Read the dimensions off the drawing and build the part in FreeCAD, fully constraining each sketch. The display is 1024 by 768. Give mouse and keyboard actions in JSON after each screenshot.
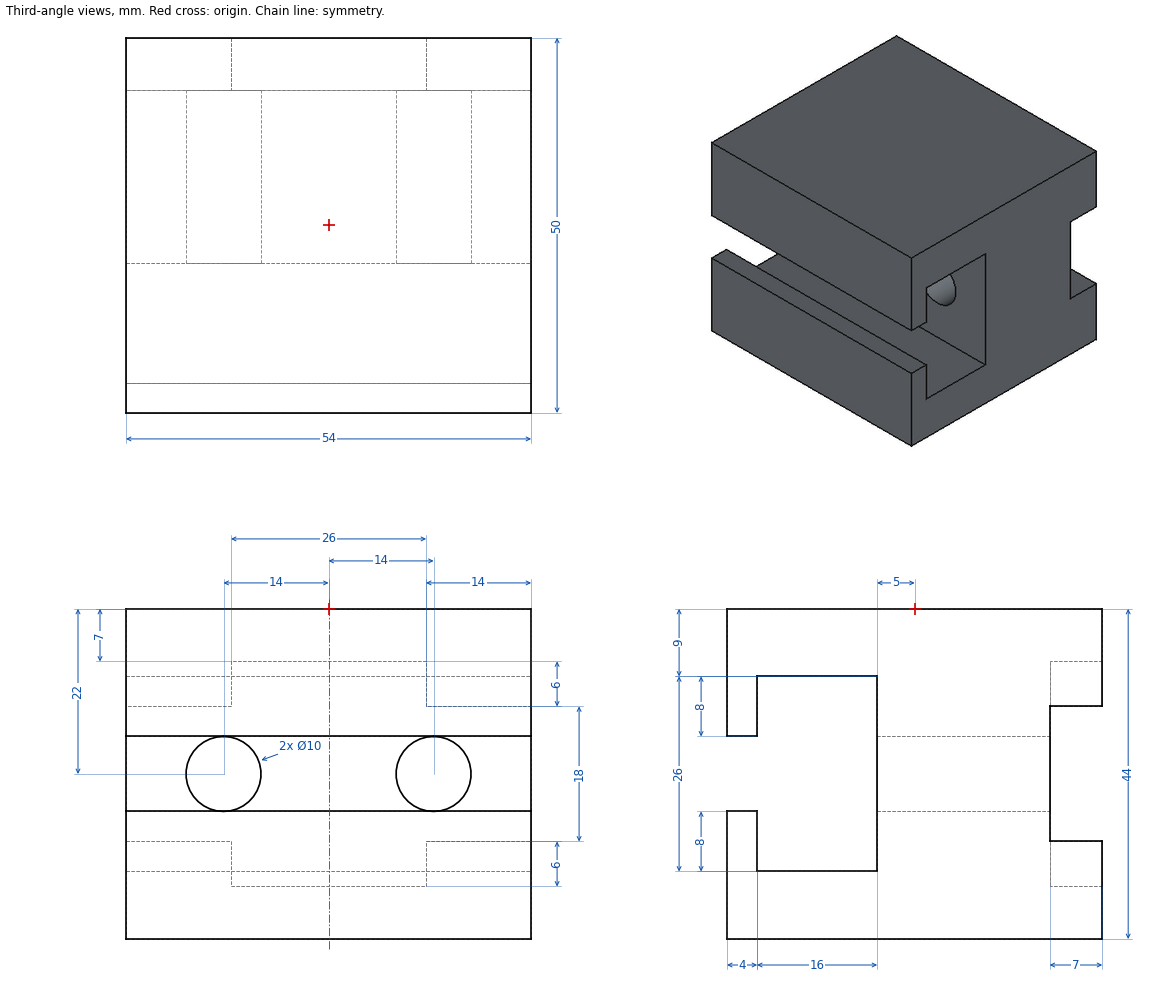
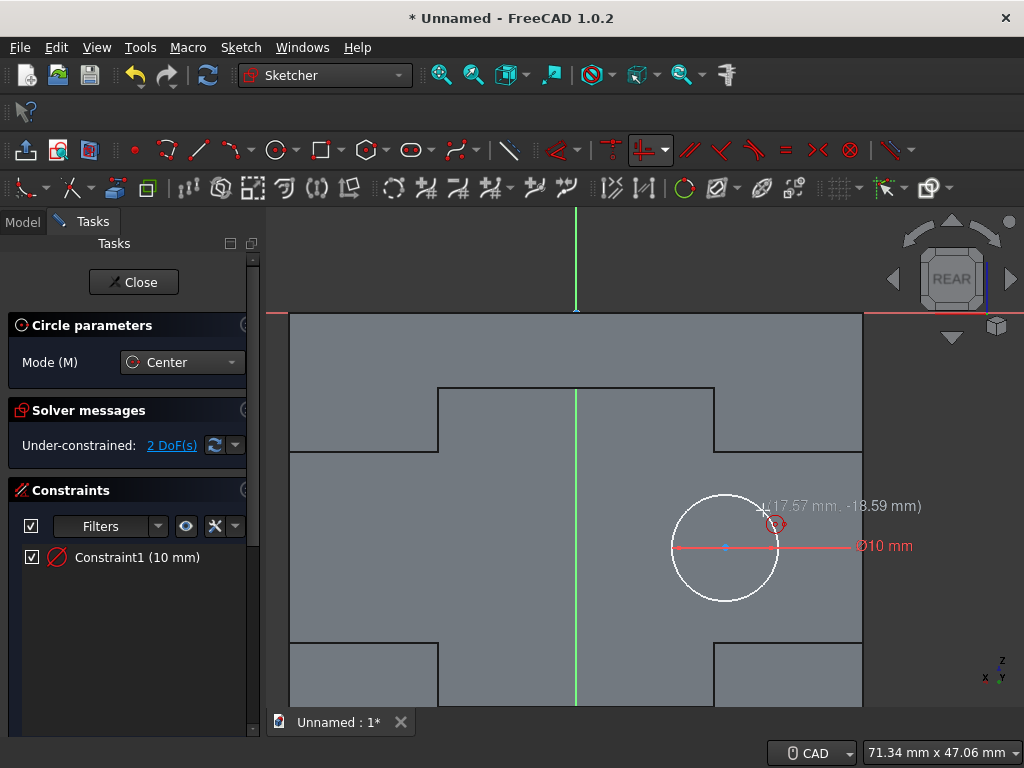
{"action": "left_click", "coordinate": [428, 547]}
{"action": "mouse_move", "coordinate": [465, 510]}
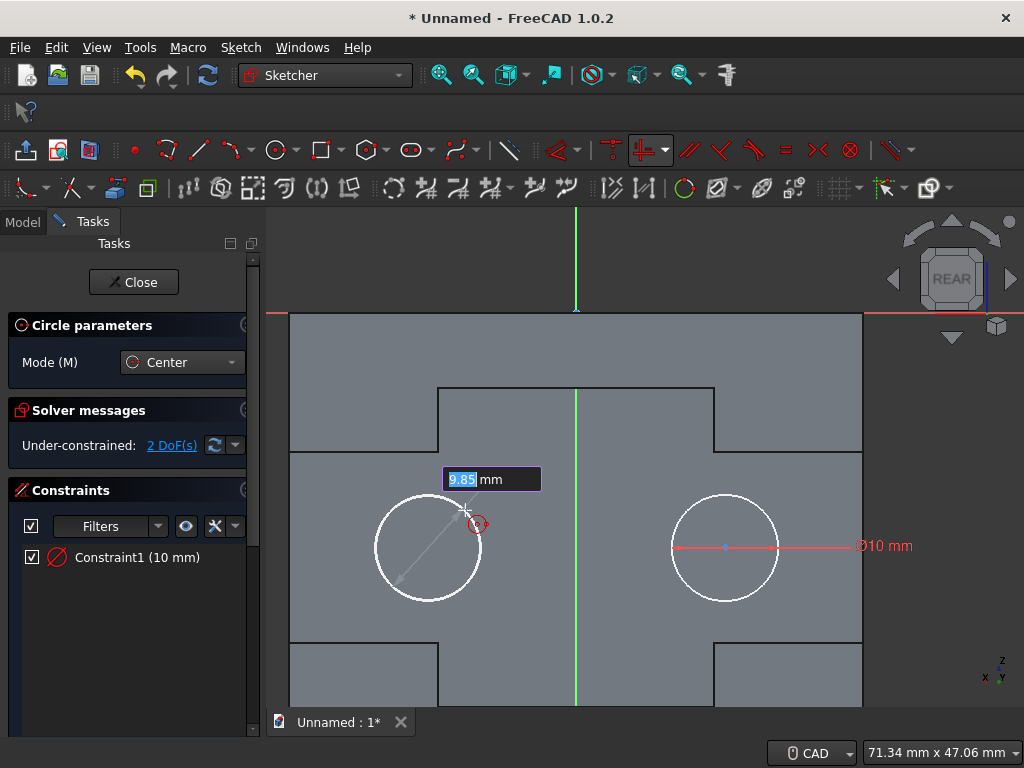
{"action": "type", "text": "10"}
{"action": "key", "text": "Return"}
{"action": "key", "text": "Escape"}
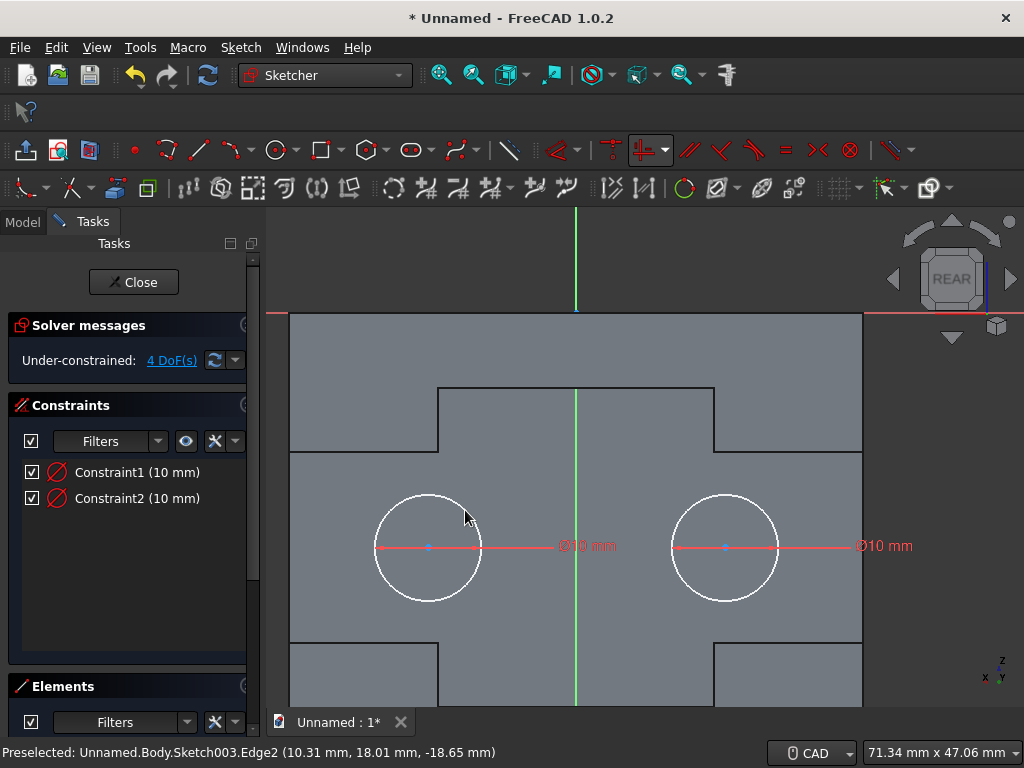
{"action": "left_click", "coordinate": [725, 548]}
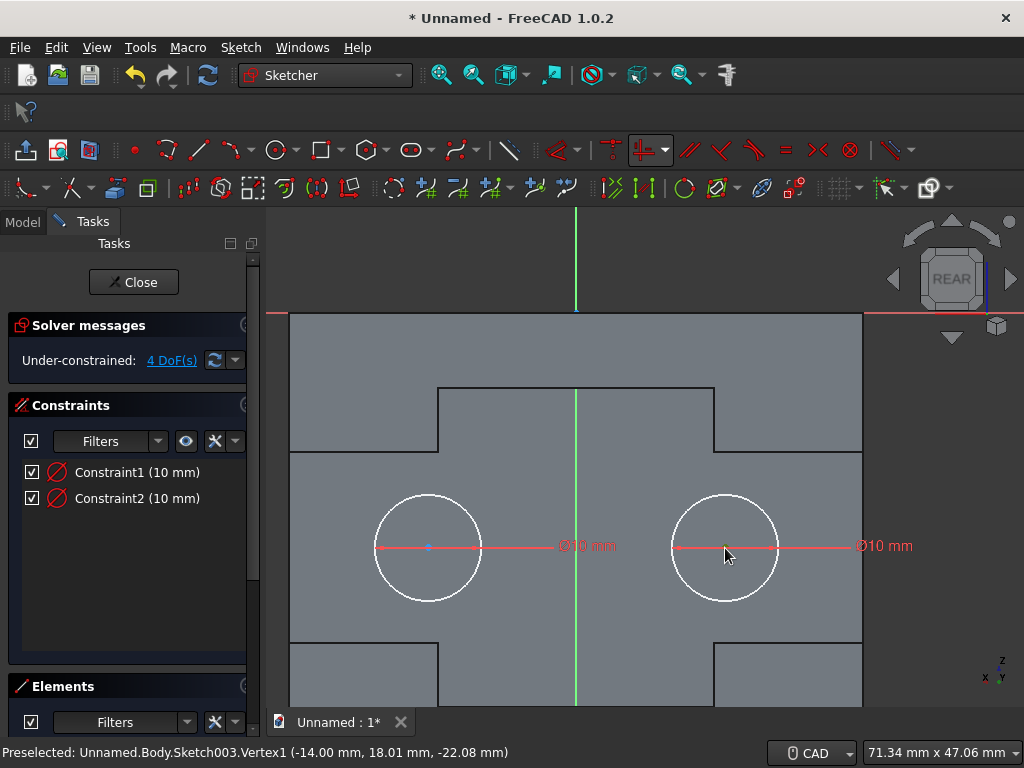
{"action": "left_click", "coordinate": [428, 548]}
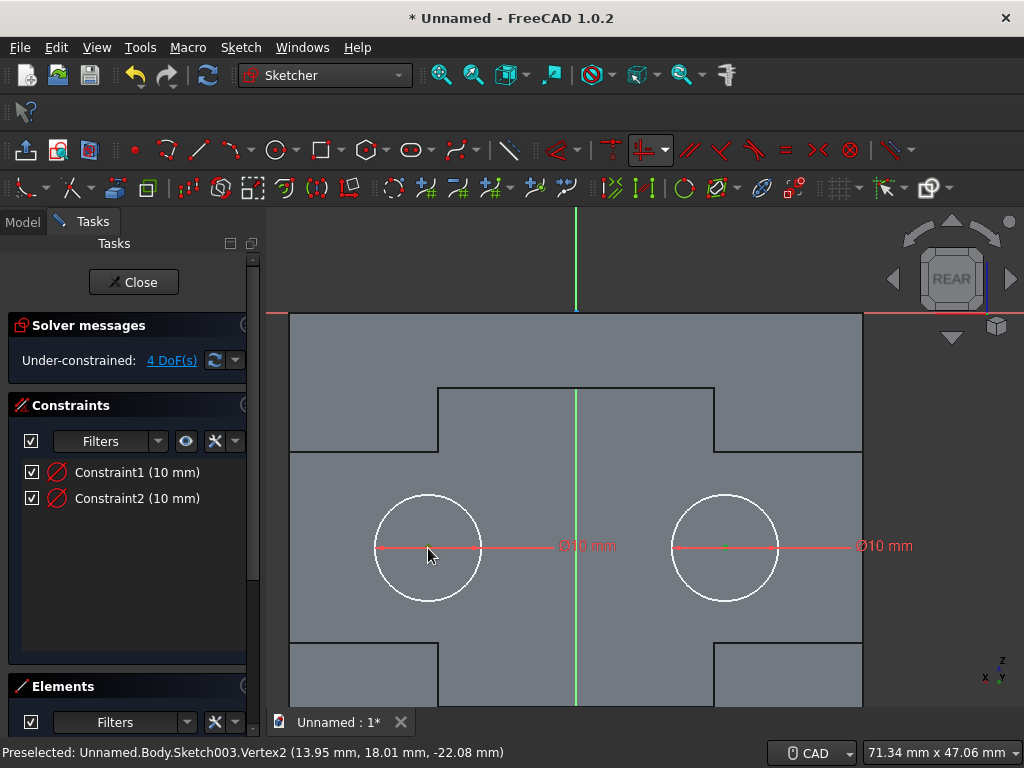
{"action": "key", "text": "h"}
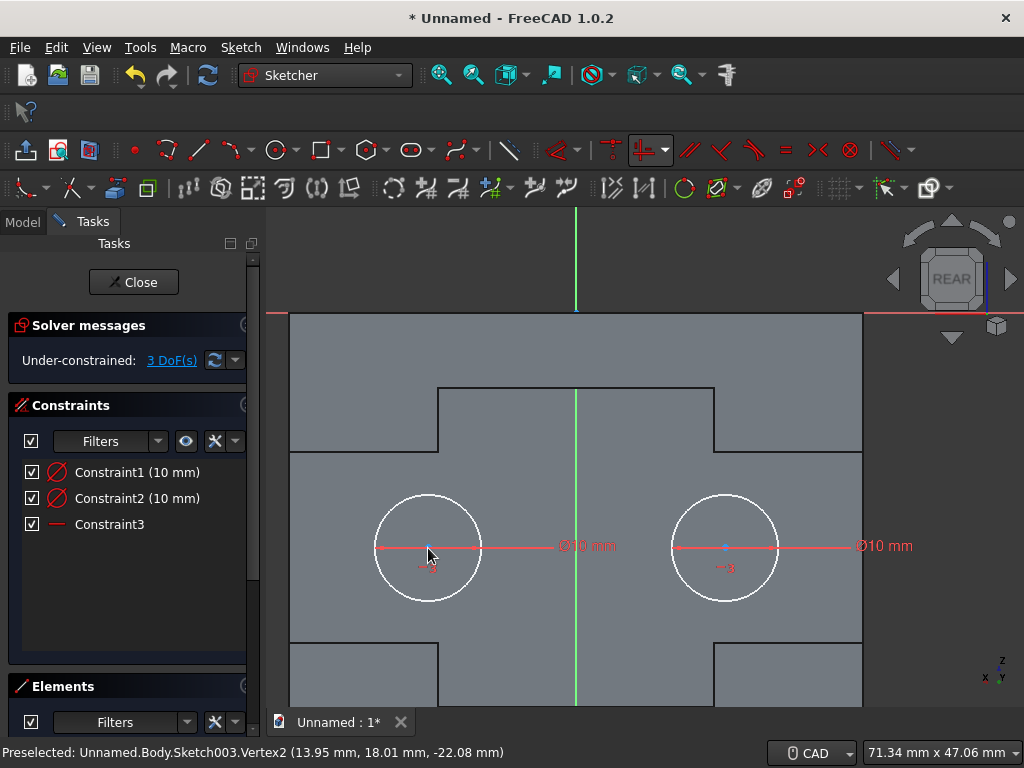
{"action": "left_click", "coordinate": [556, 150]}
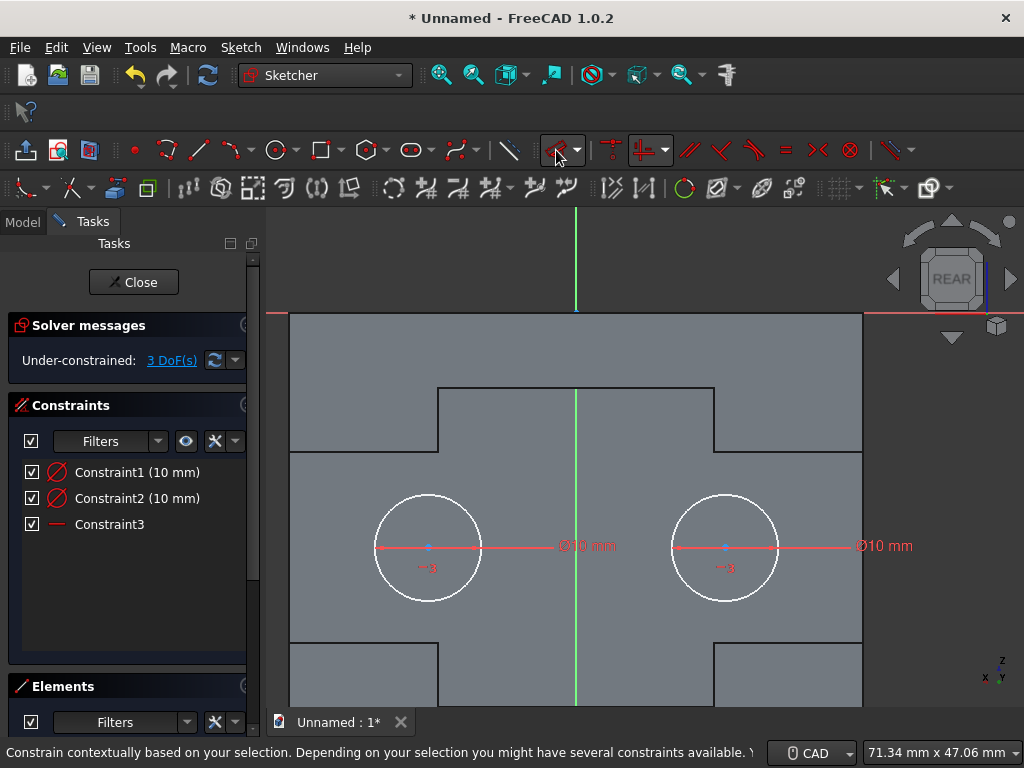
{"action": "left_click", "coordinate": [725, 548]}
{"action": "left_click", "coordinate": [651, 279]}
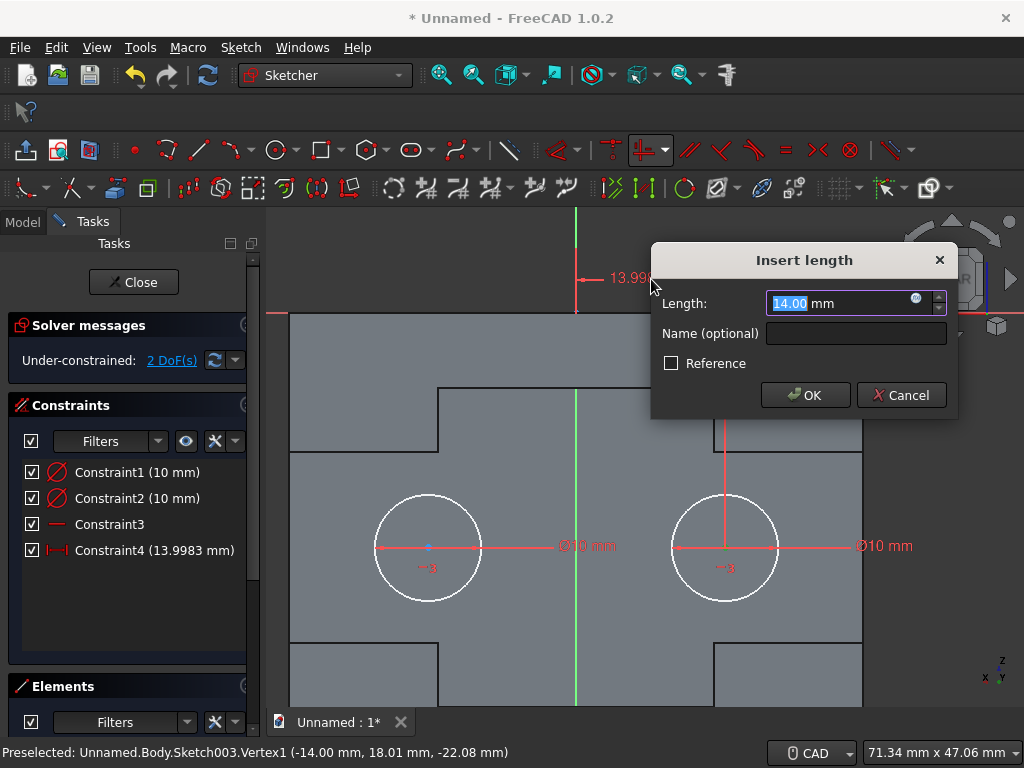
{"action": "type", "text": "14"}
{"action": "key", "text": "Return"}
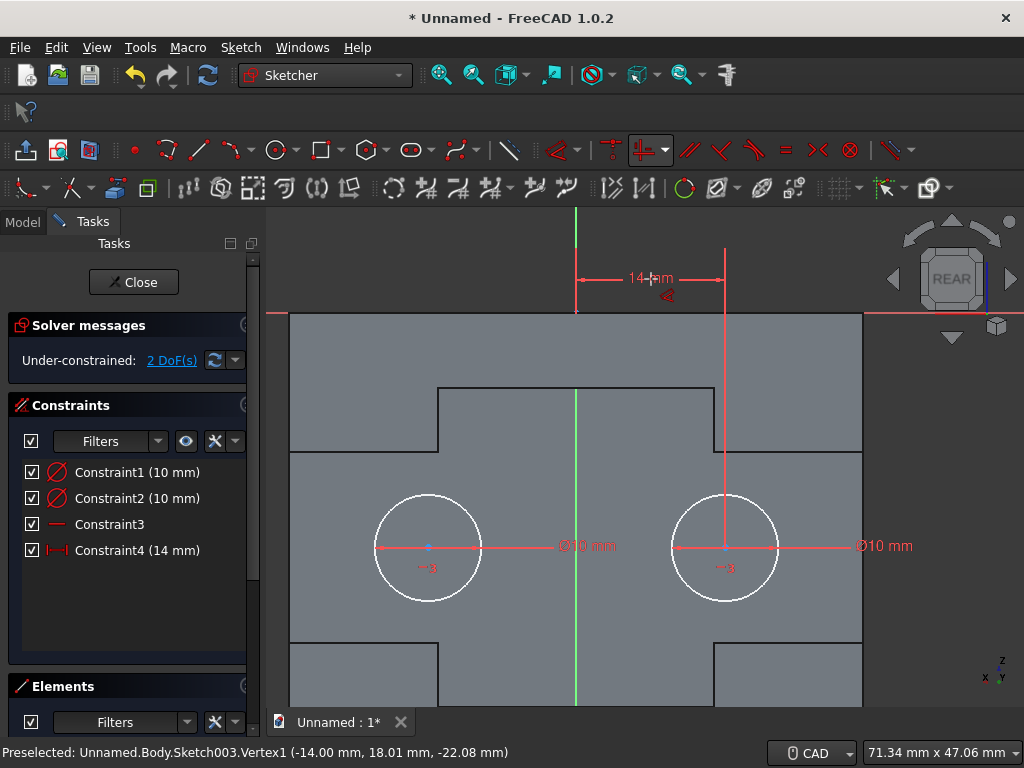
{"action": "left_click", "coordinate": [725, 548]}
{"action": "left_click", "coordinate": [759, 431]}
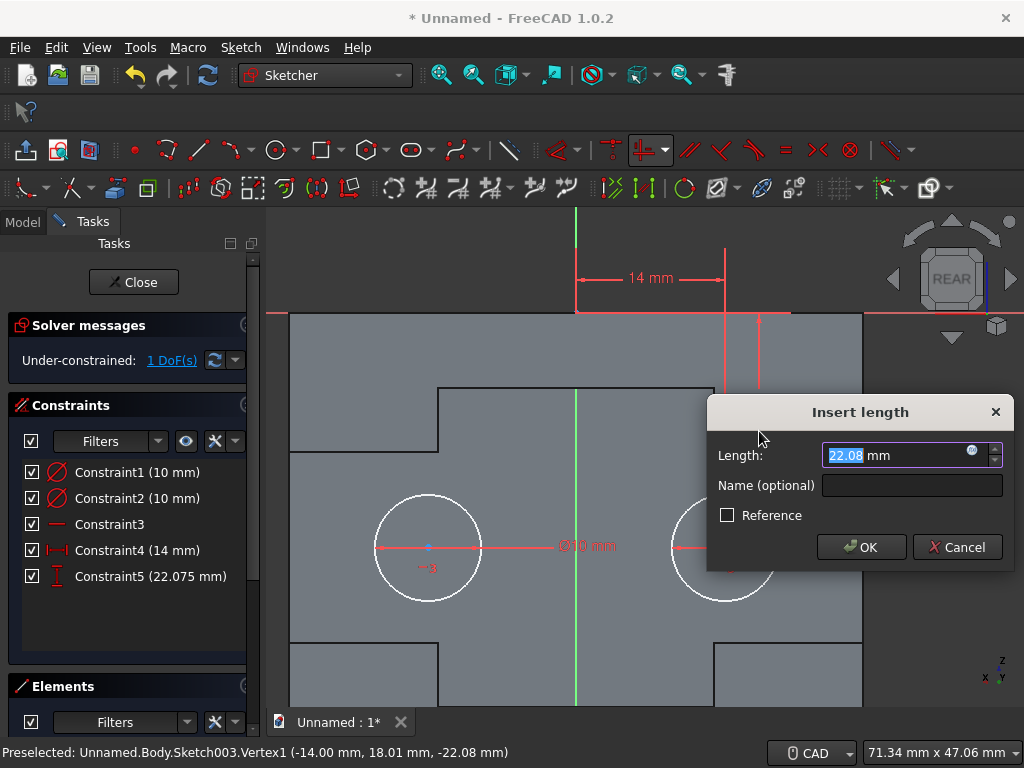
{"action": "type", "text": "22"}
{"action": "key", "text": "Return"}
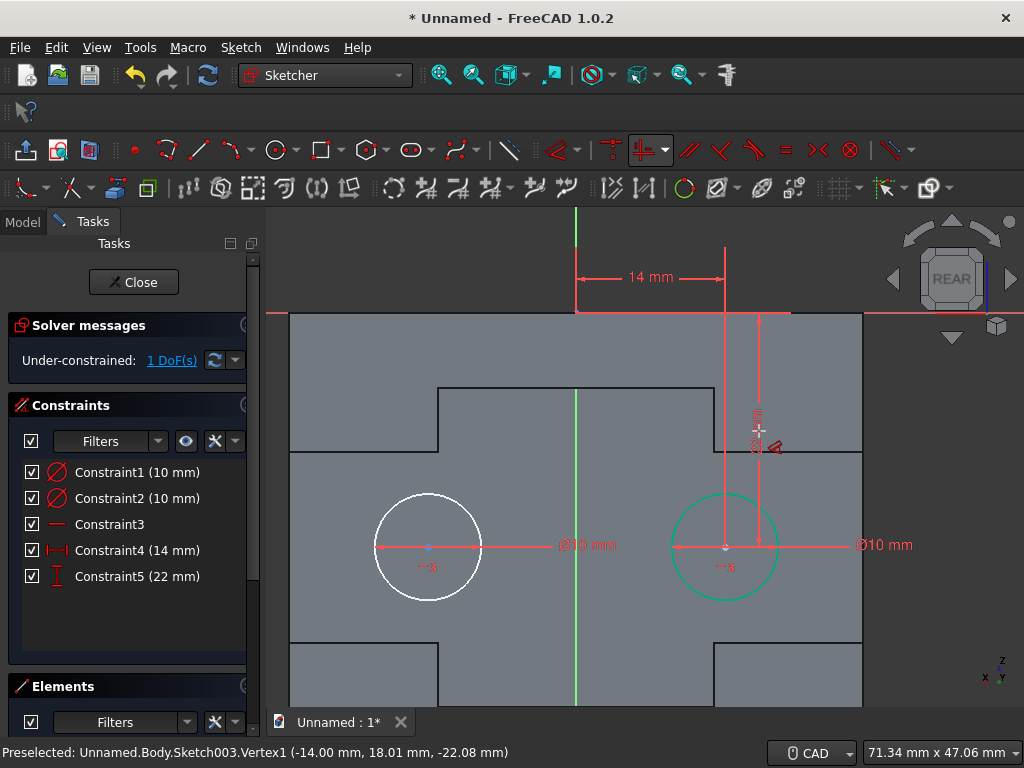
{"action": "left_click", "coordinate": [428, 547]}
{"action": "left_click", "coordinate": [502, 279]}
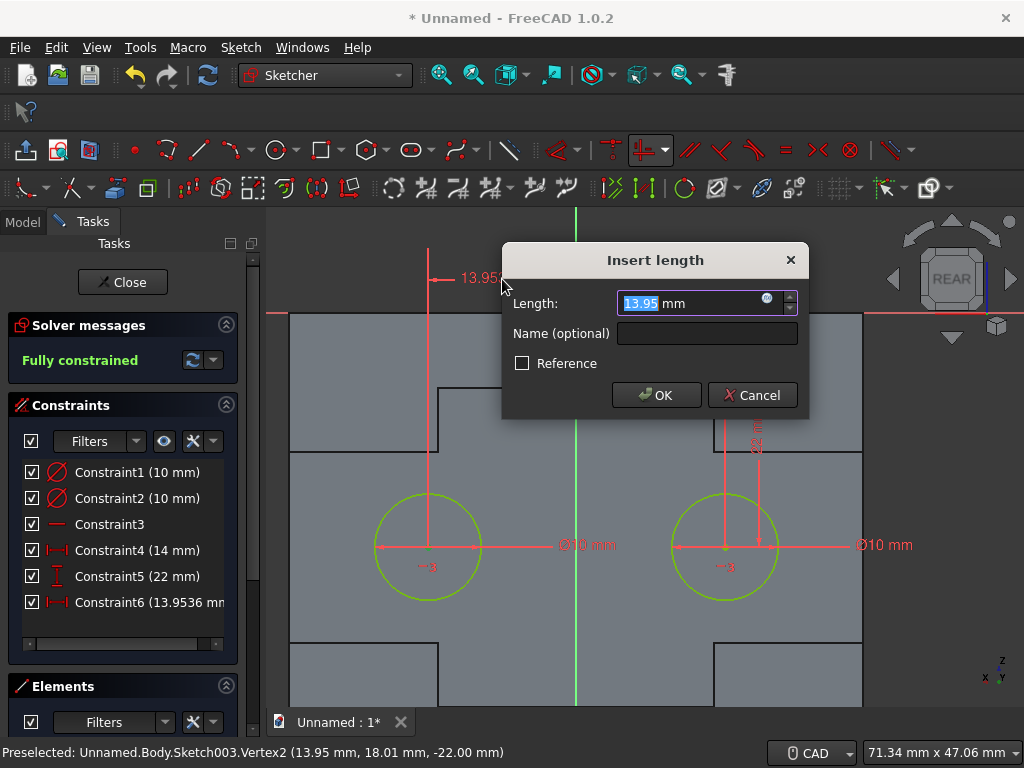
{"action": "type", "text": "14"}
{"action": "key", "text": "Return"}
{"action": "key", "text": "Escape"}